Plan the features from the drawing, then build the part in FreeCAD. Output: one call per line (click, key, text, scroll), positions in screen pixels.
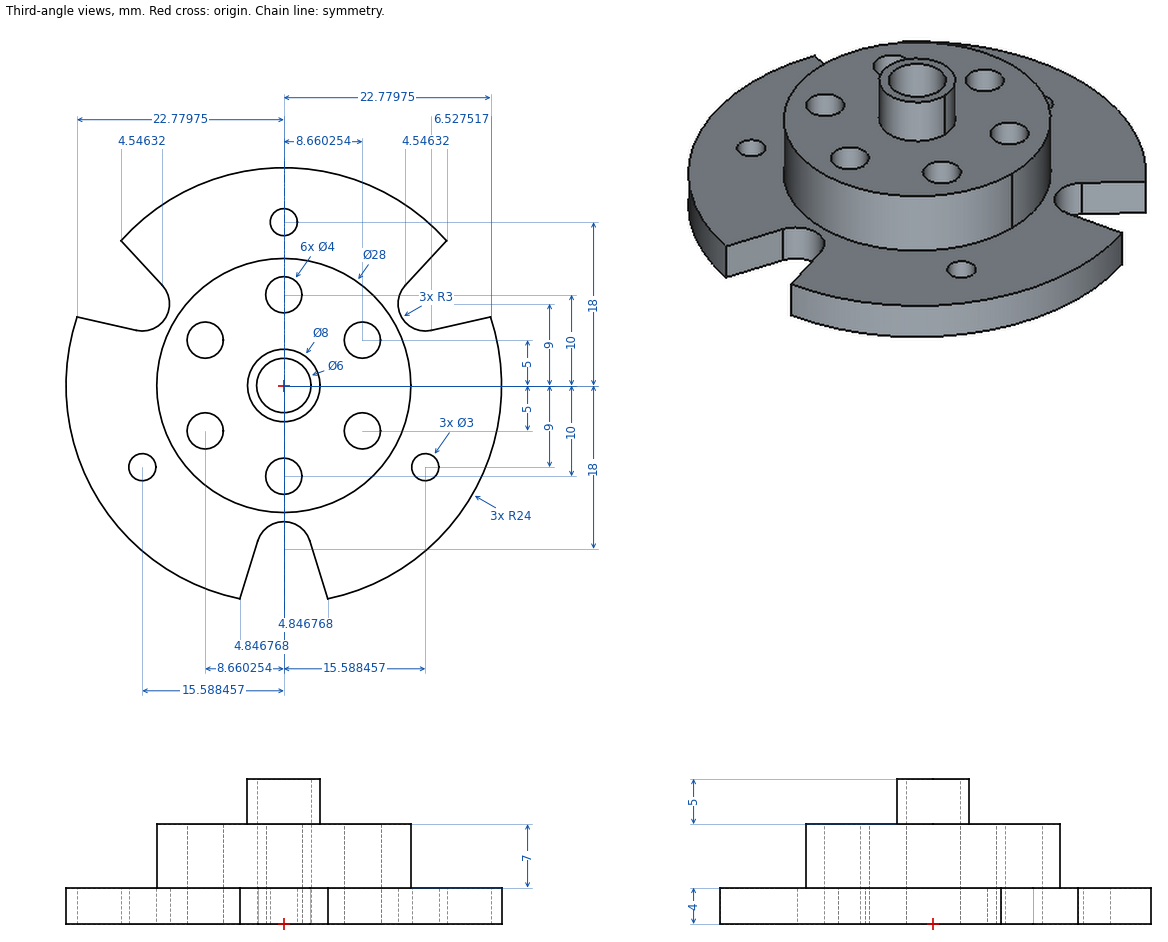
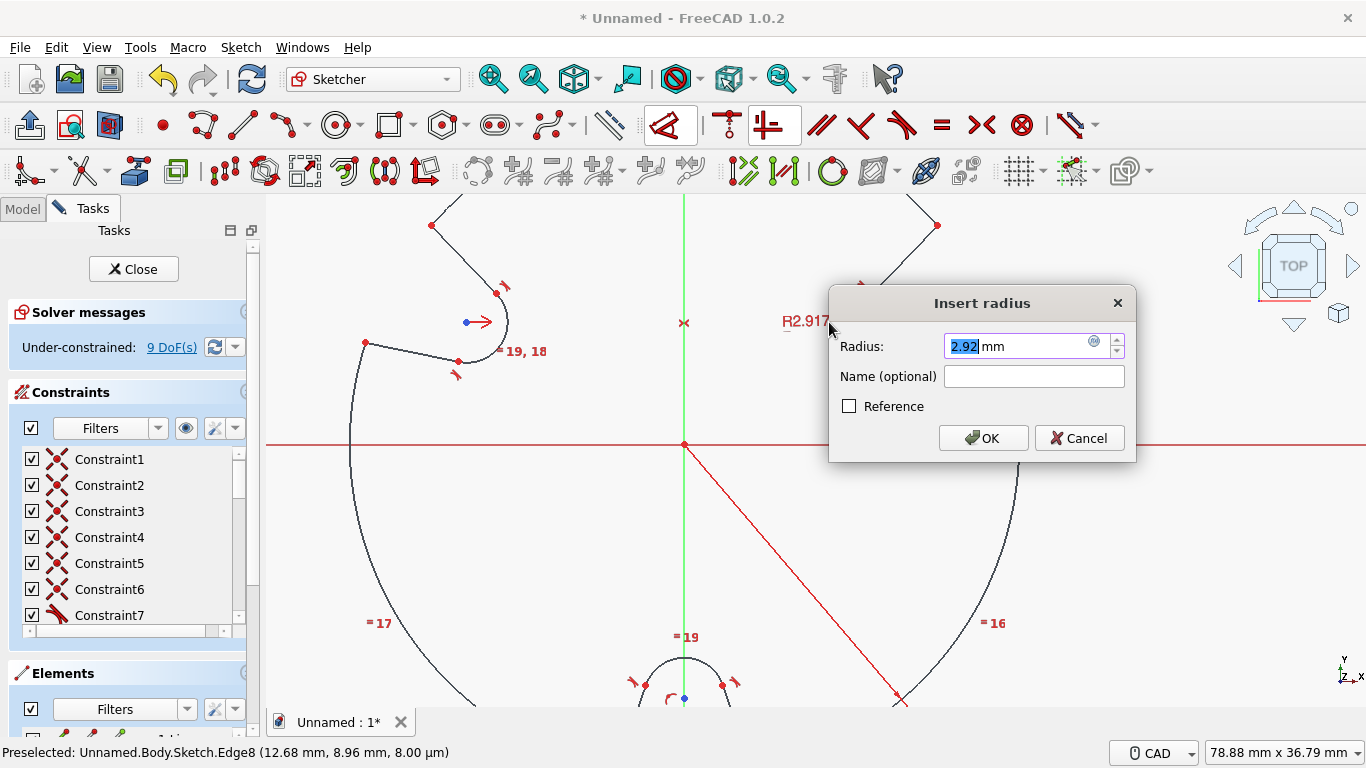
text(3)
key(Return)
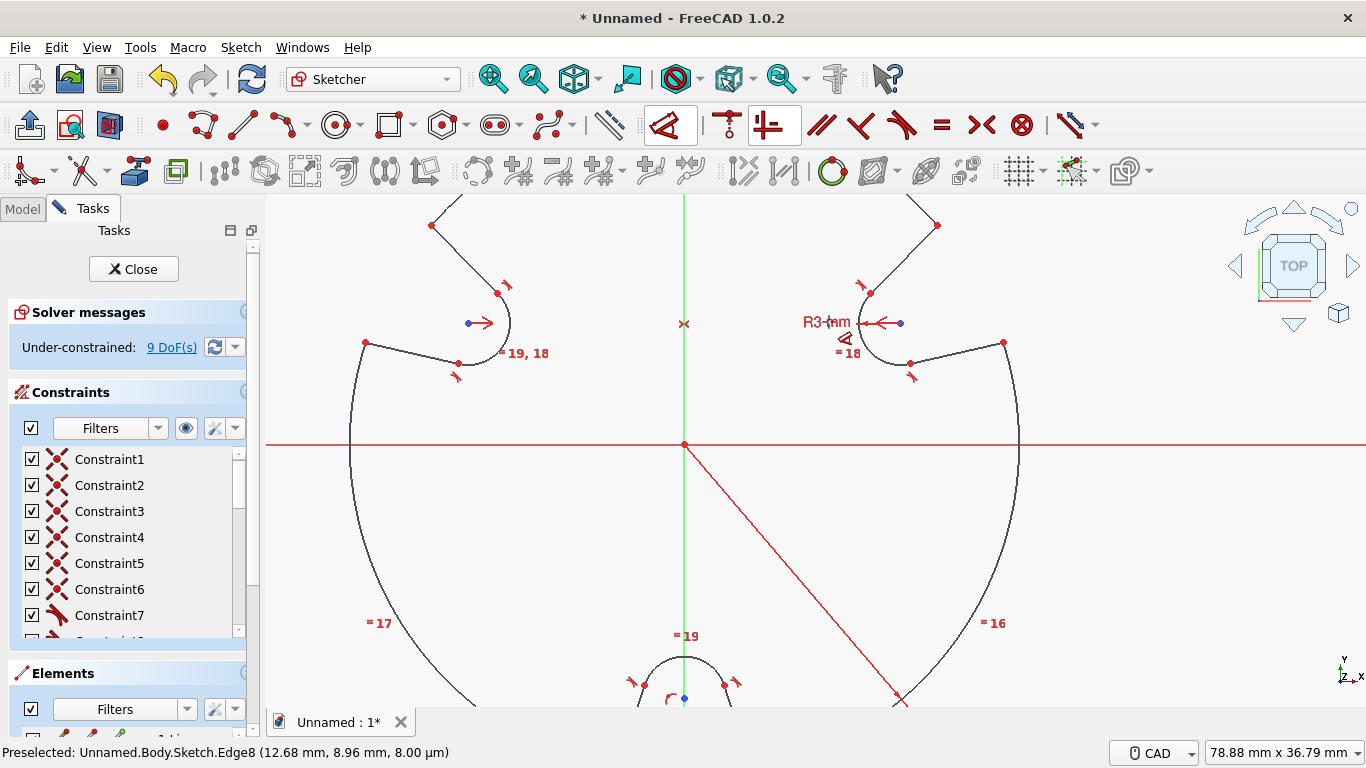
click(901, 323)
click(935, 384)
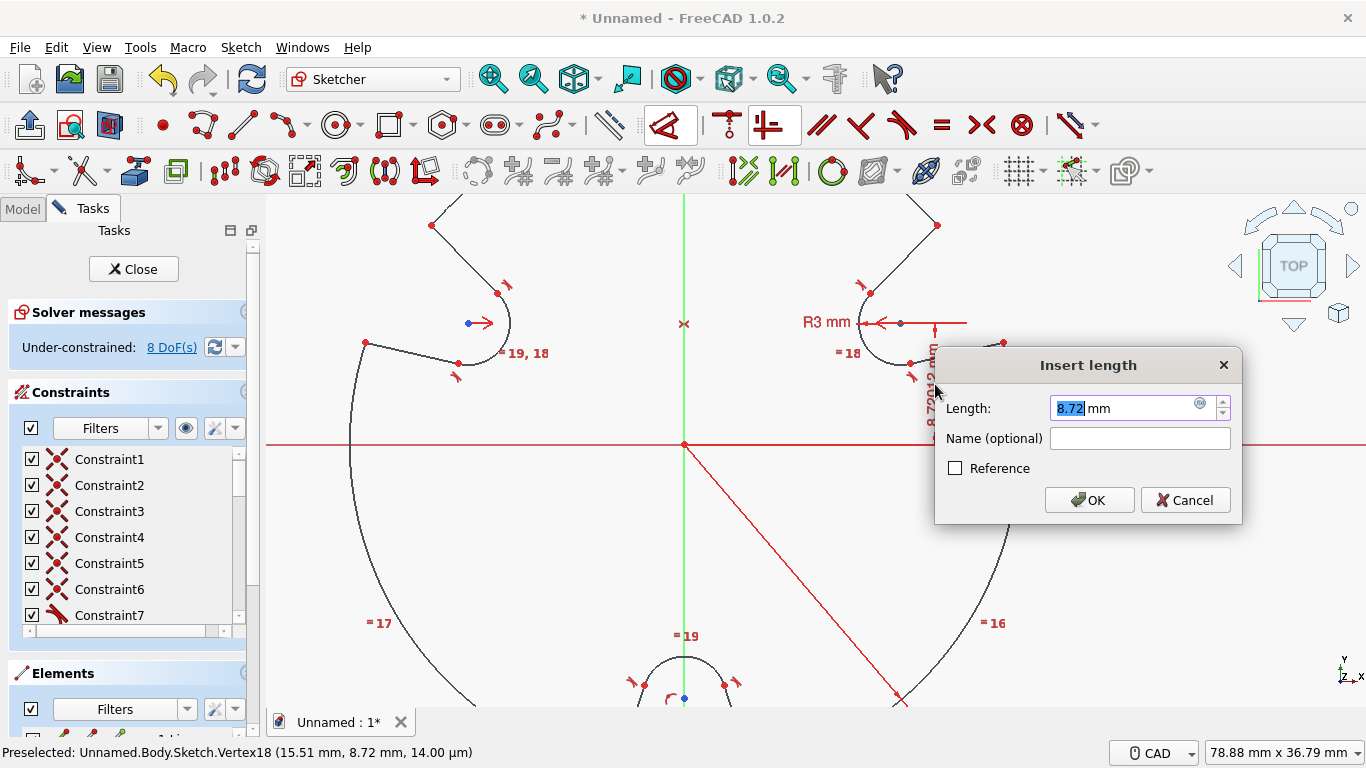
text(9)
key(Return)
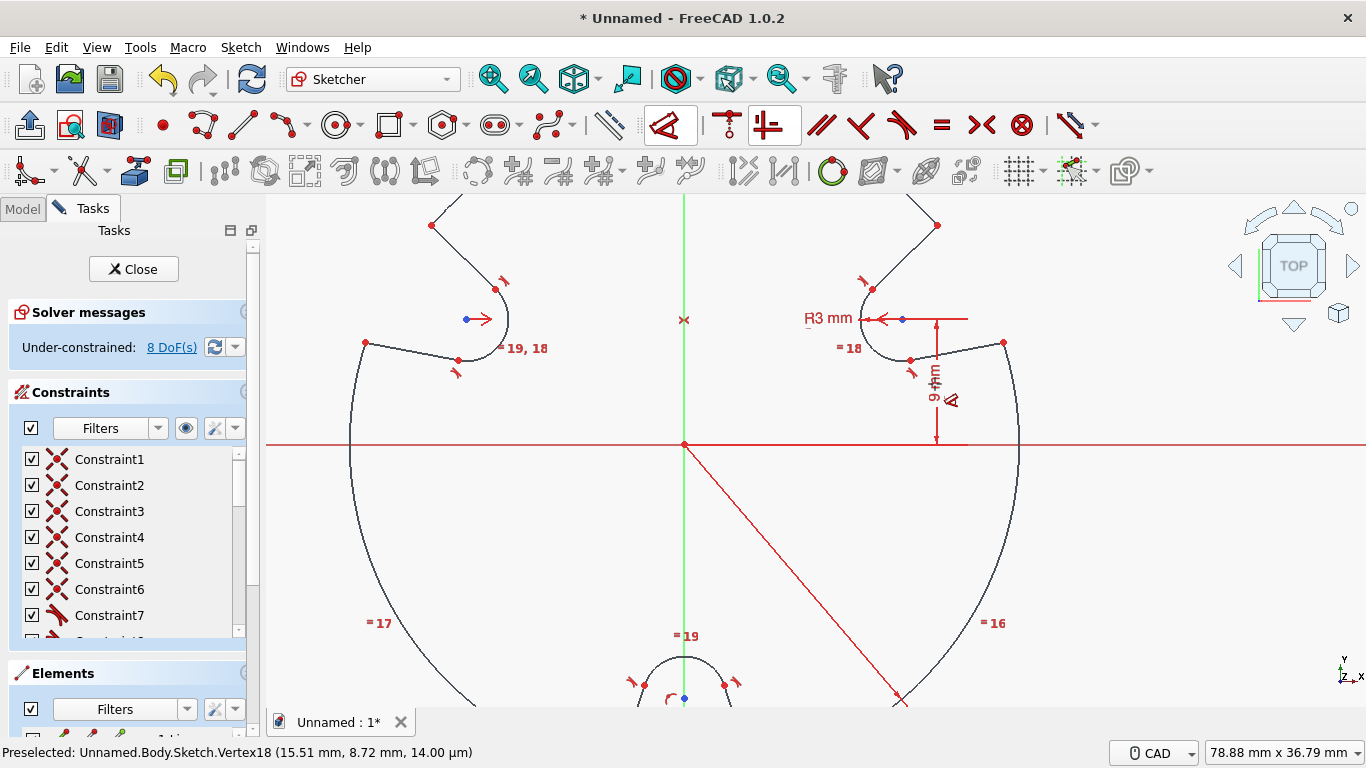
scroll(799, 458, down, 4)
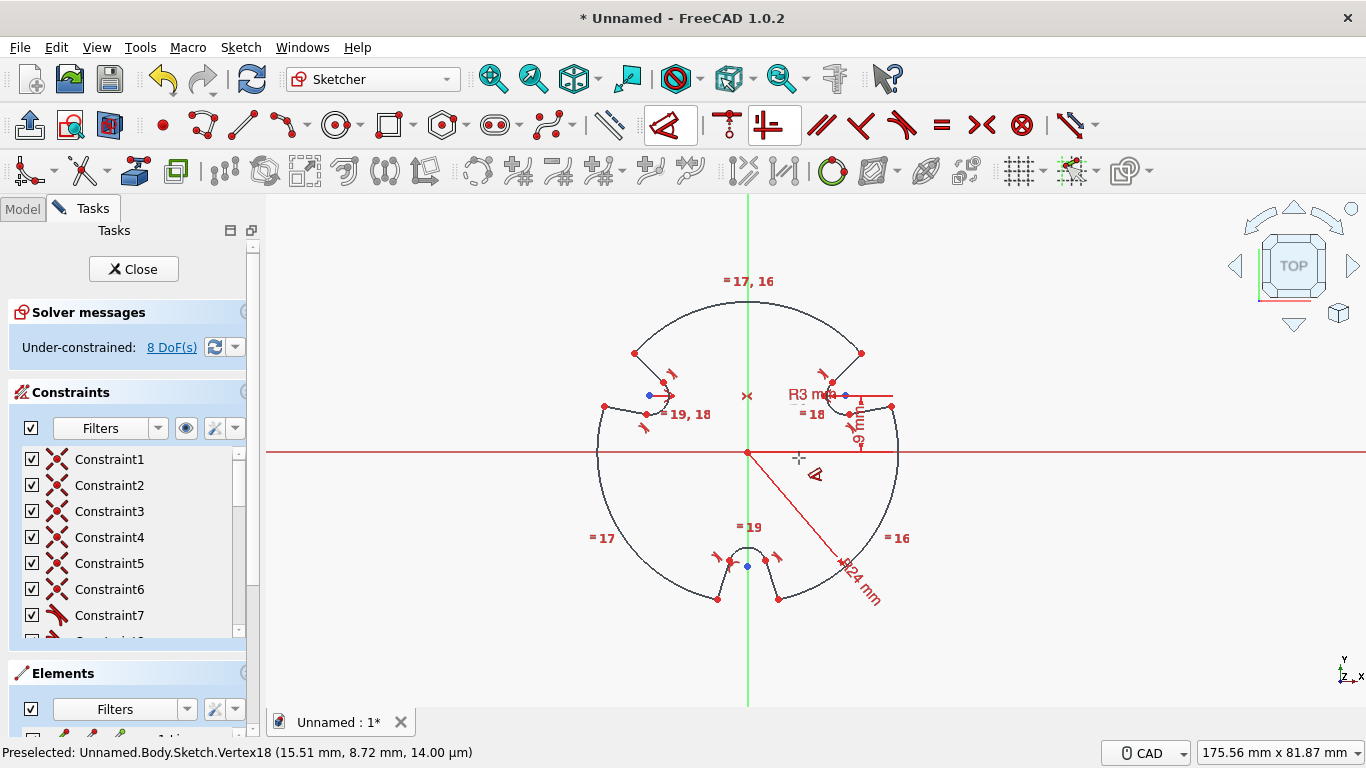
click(748, 566)
click(782, 509)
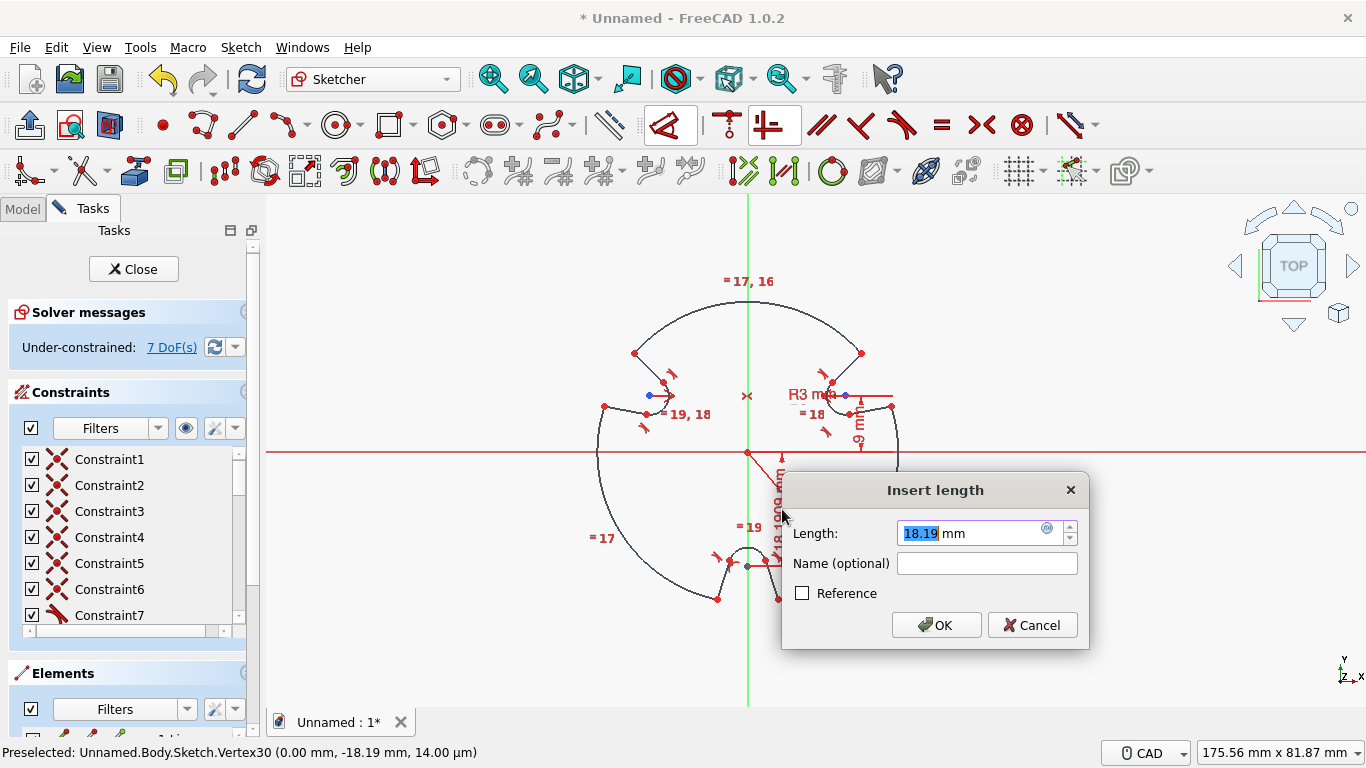
text(18)
key(Return)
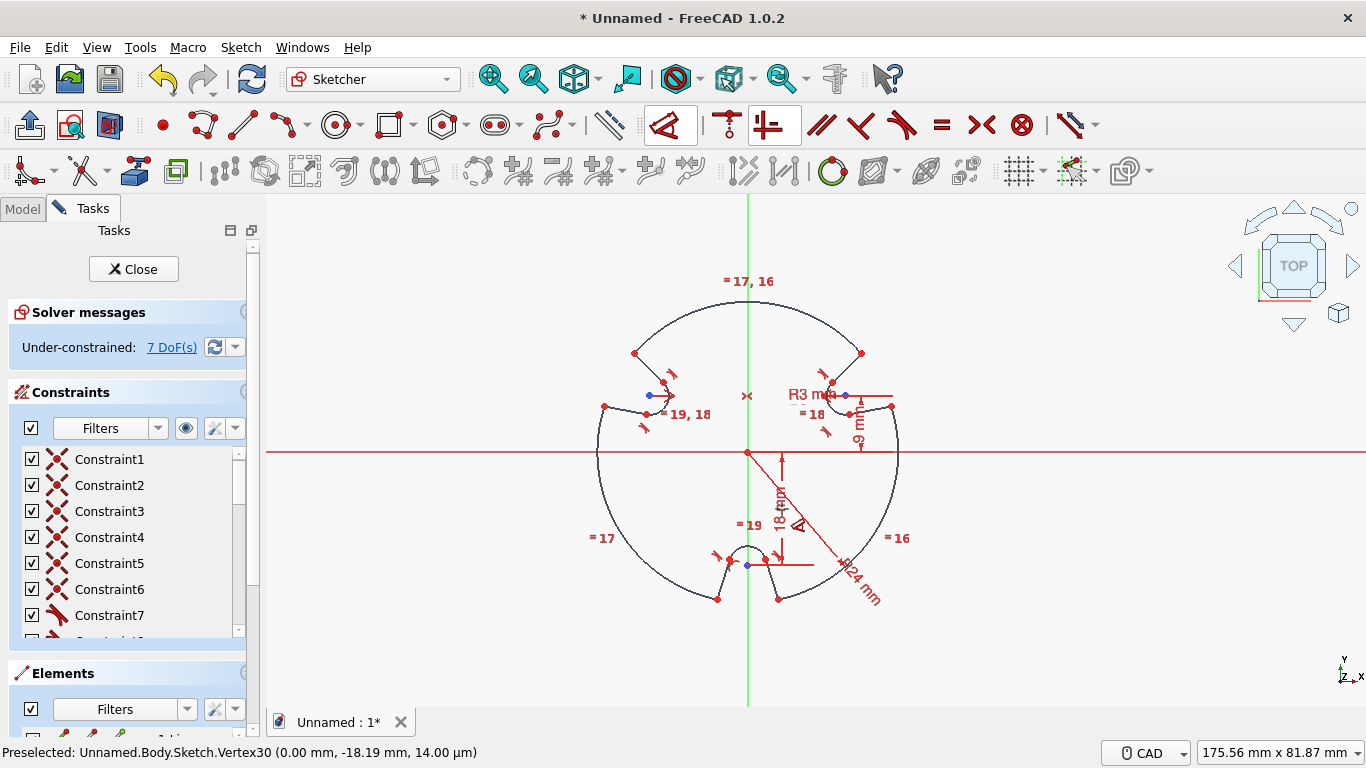
scroll(841, 374, up, 2)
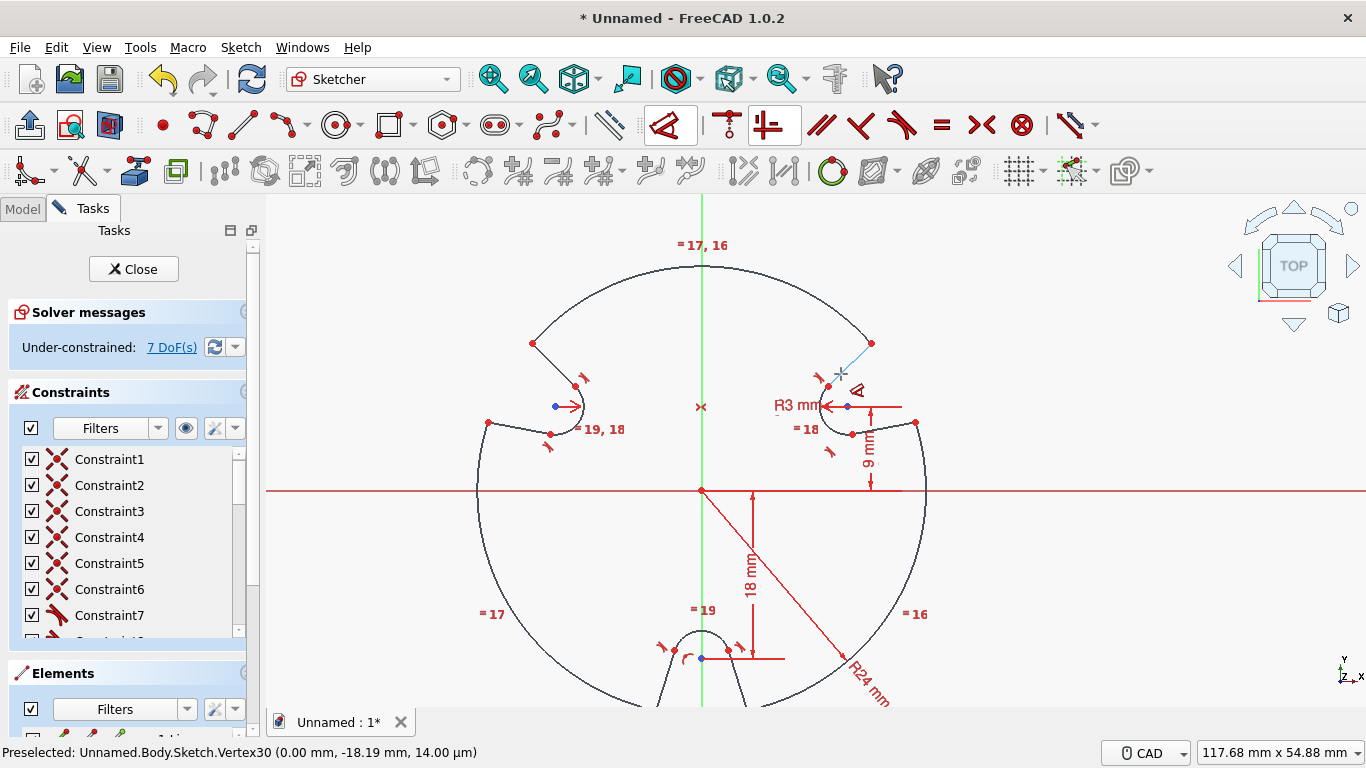
click(841, 374)
click(860, 310)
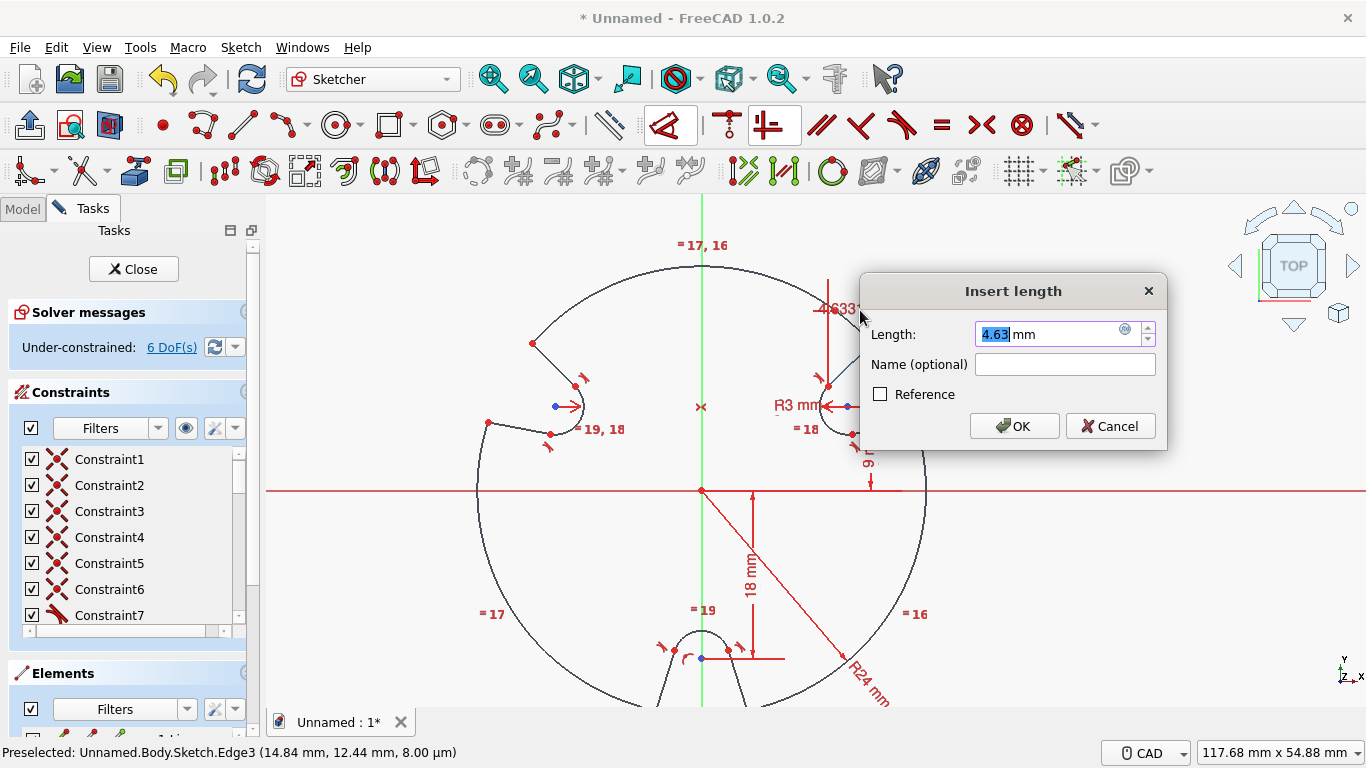
text(4.54632)
key(Return)